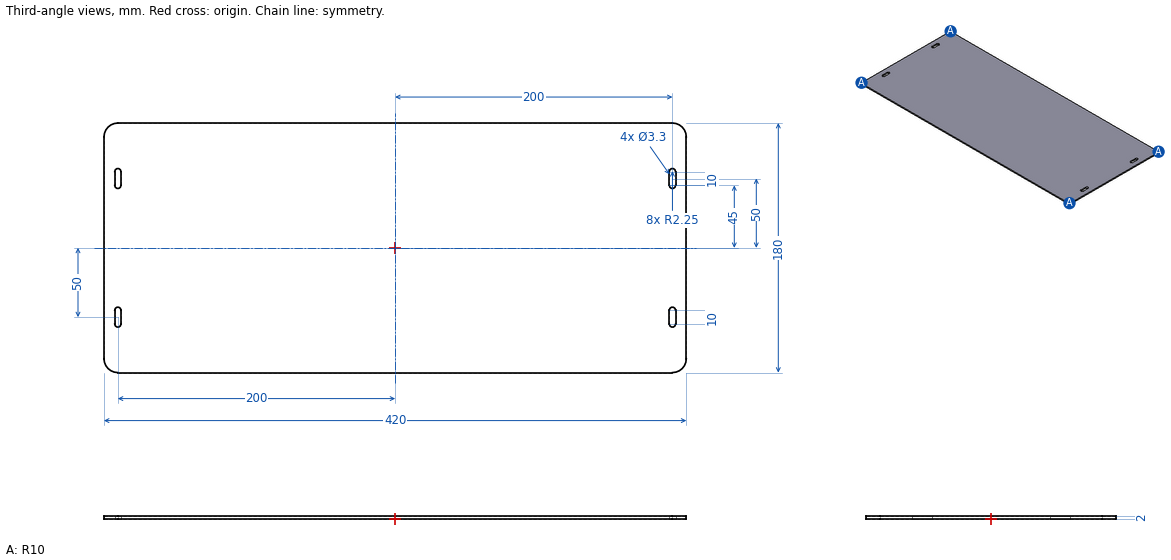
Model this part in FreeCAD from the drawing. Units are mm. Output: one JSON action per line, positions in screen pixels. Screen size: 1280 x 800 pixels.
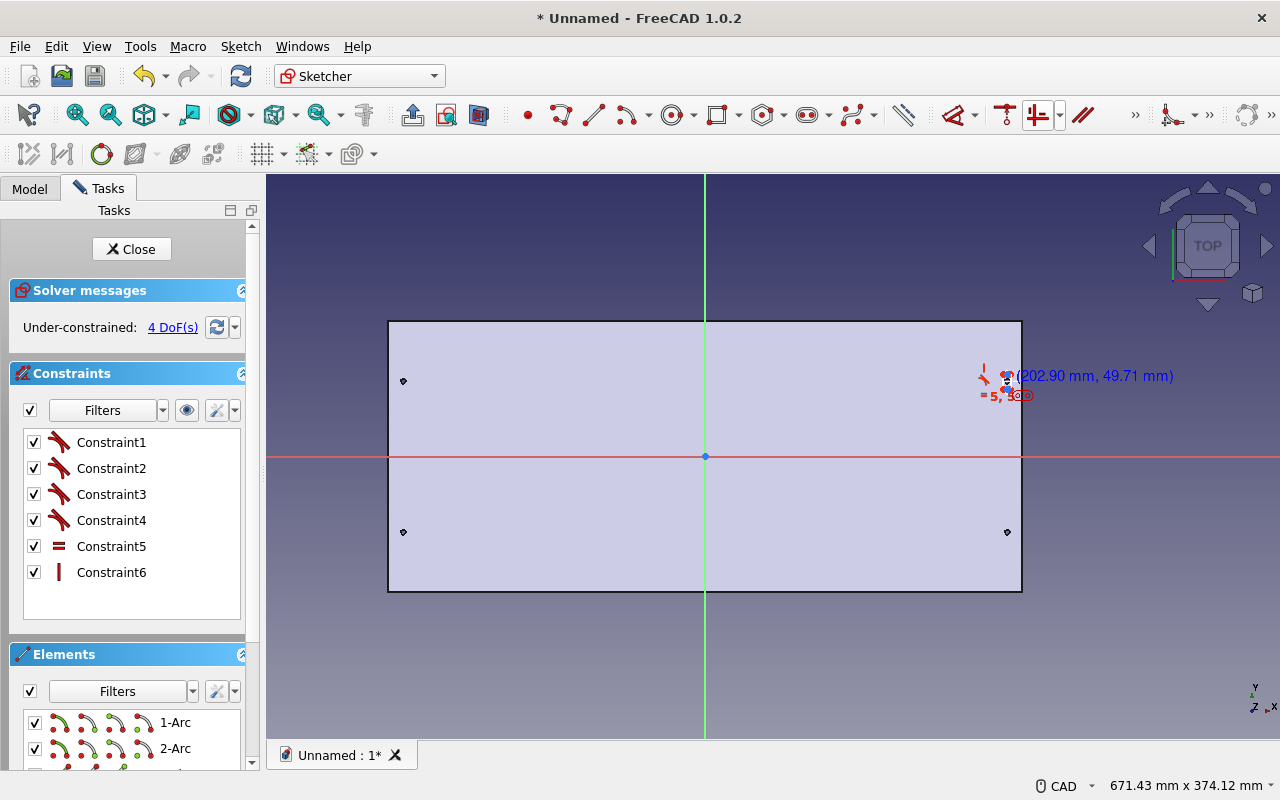
{"action": "scroll", "coordinate": [1007, 540], "scroll_direction": "up", "scroll_amount": 10}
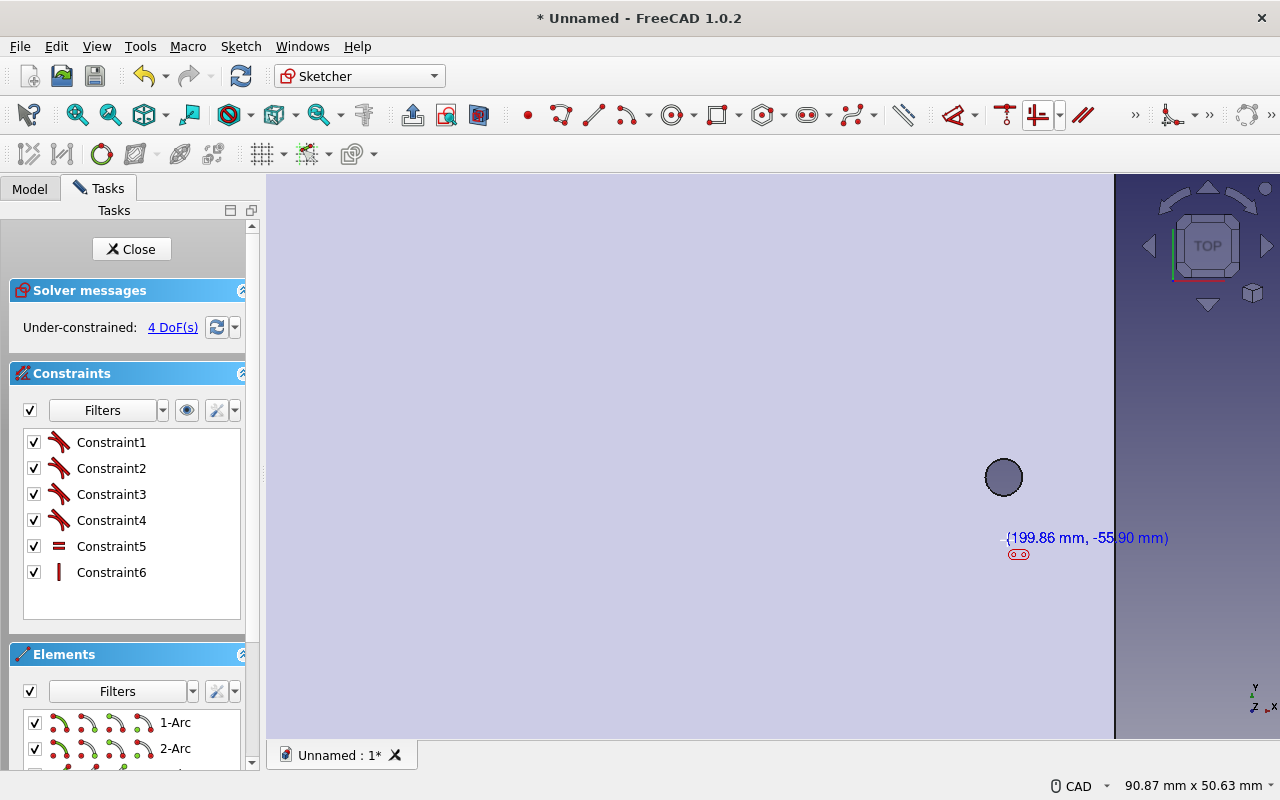
{"action": "scroll", "coordinate": [1007, 541], "scroll_direction": "down", "scroll_amount": 10}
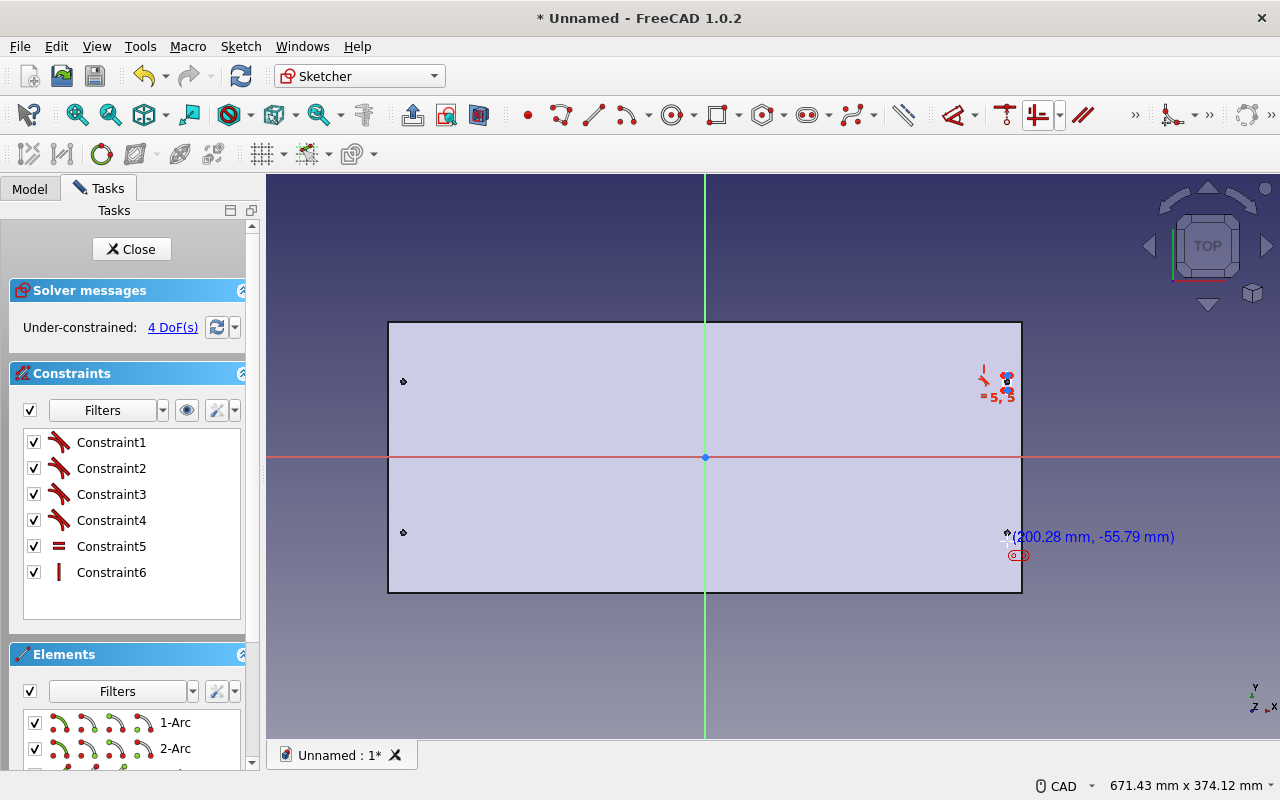
{"action": "left_click", "coordinate": [1007, 540]}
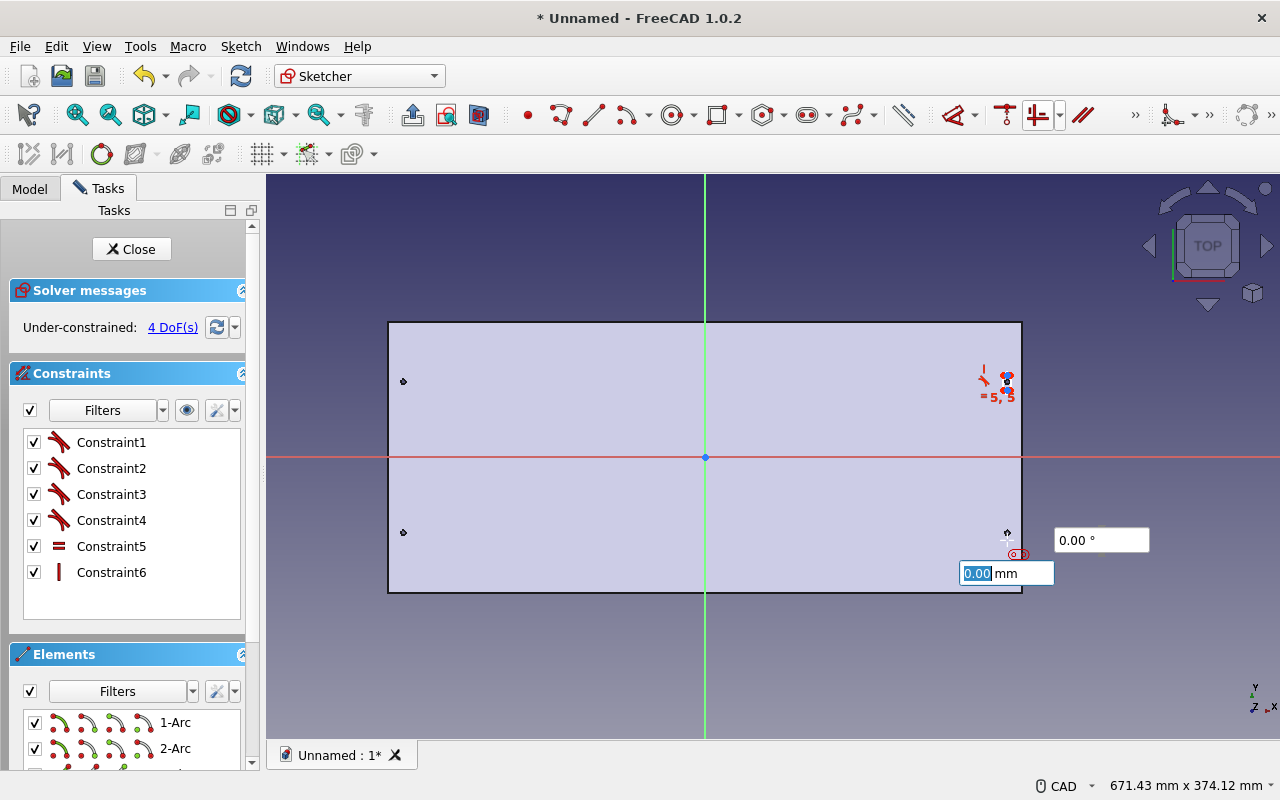
{"action": "left_click", "coordinate": [1007, 525]}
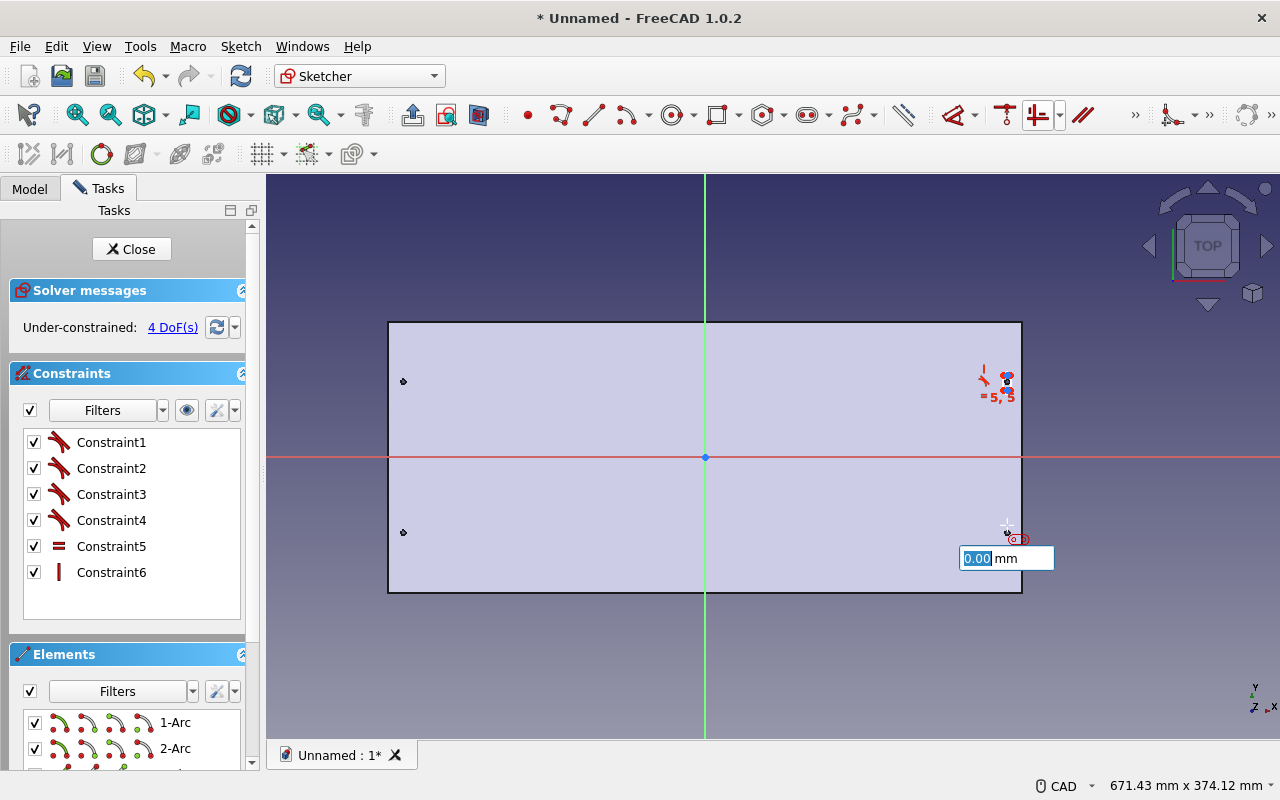
{"action": "scroll", "coordinate": [1004, 533], "scroll_direction": "up", "scroll_amount": 8}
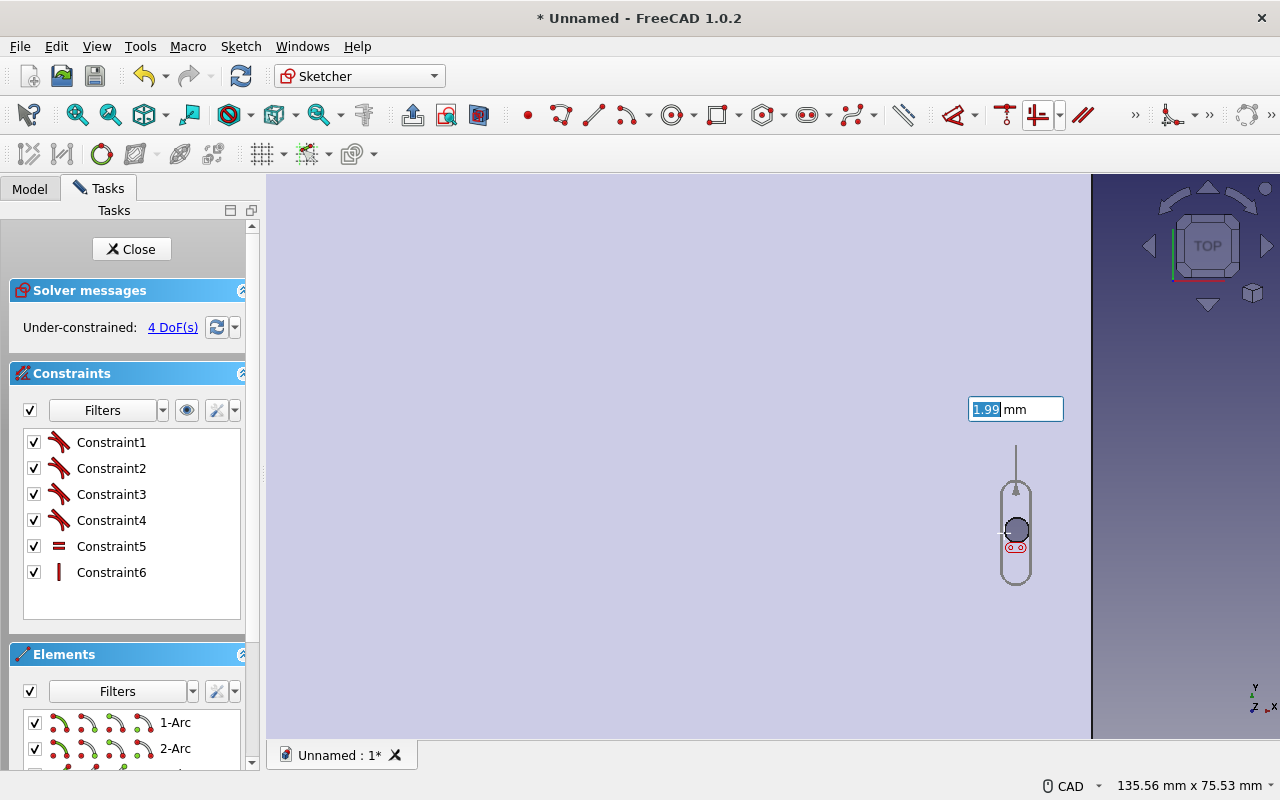
{"action": "left_click", "coordinate": [1000, 530]}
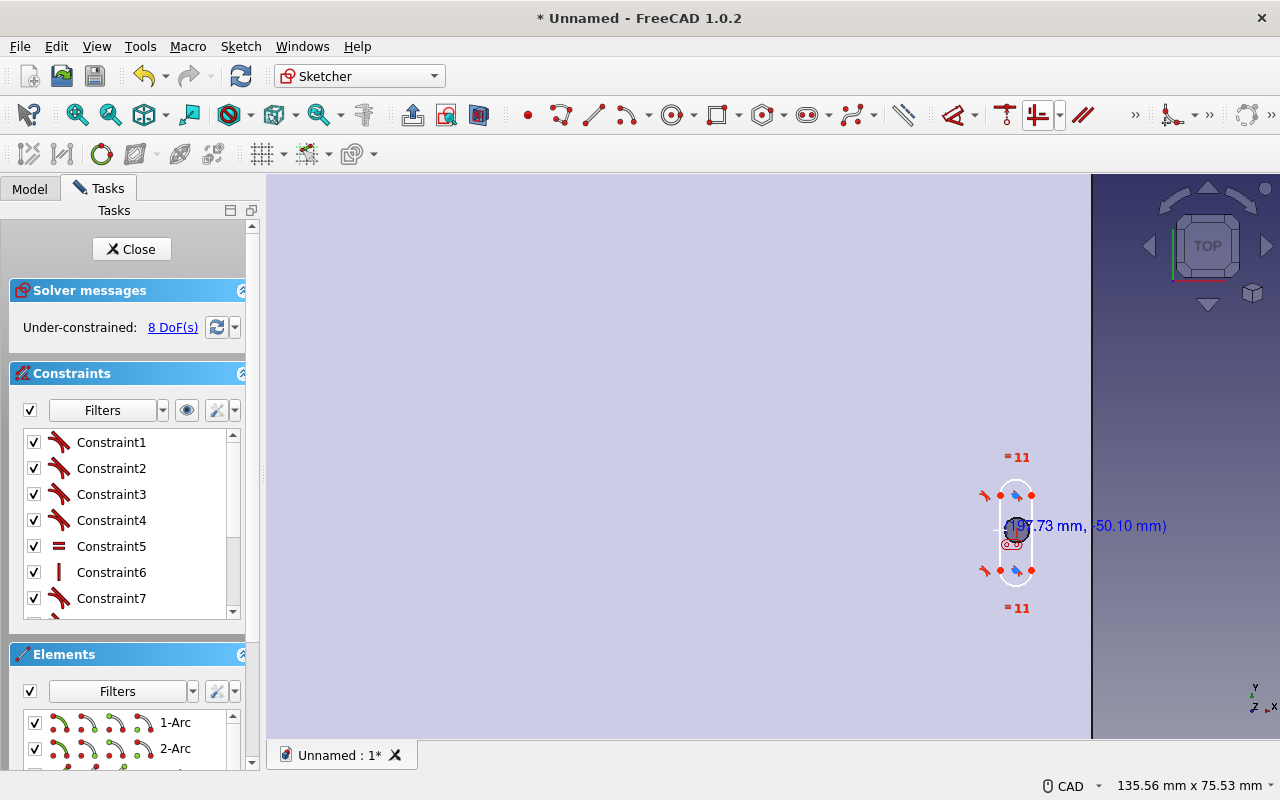
{"action": "scroll", "coordinate": [1004, 532], "scroll_direction": "down", "scroll_amount": 8}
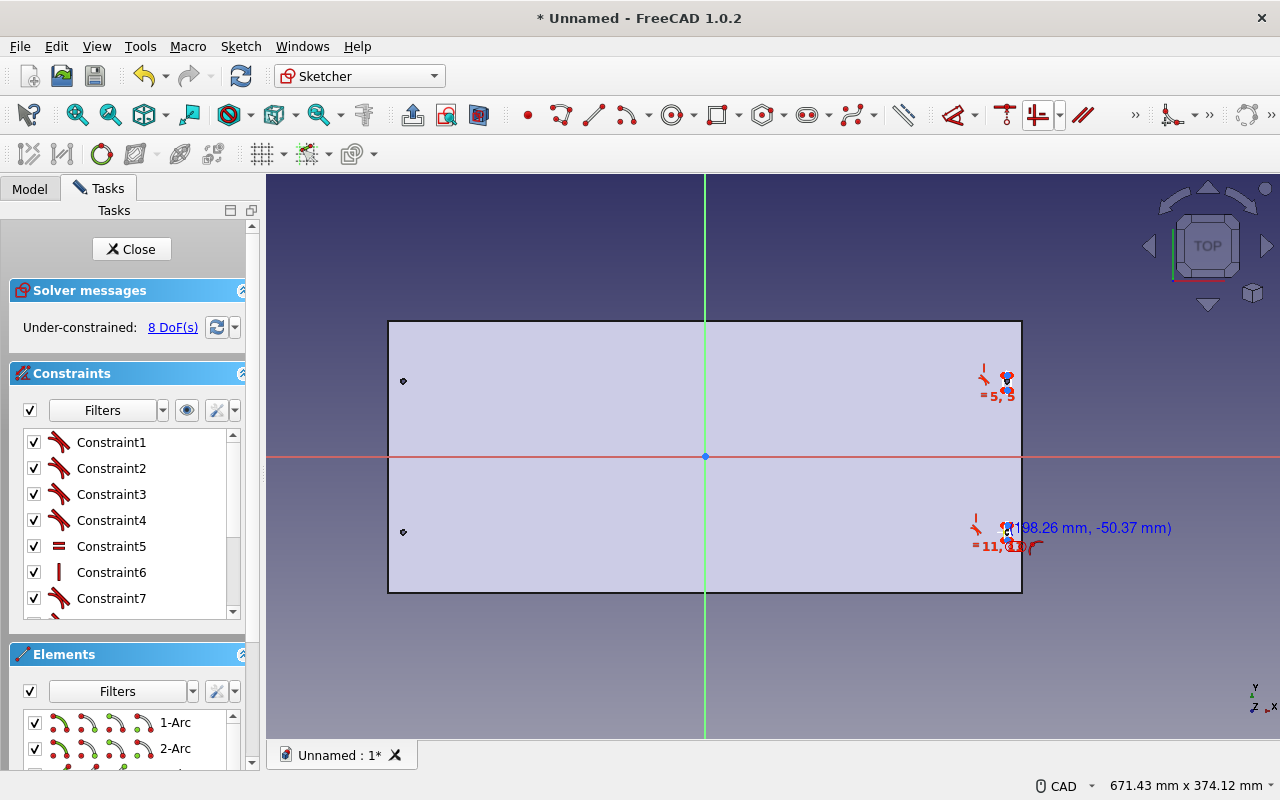
{"action": "scroll", "coordinate": [403, 540], "scroll_direction": "up", "scroll_amount": 10}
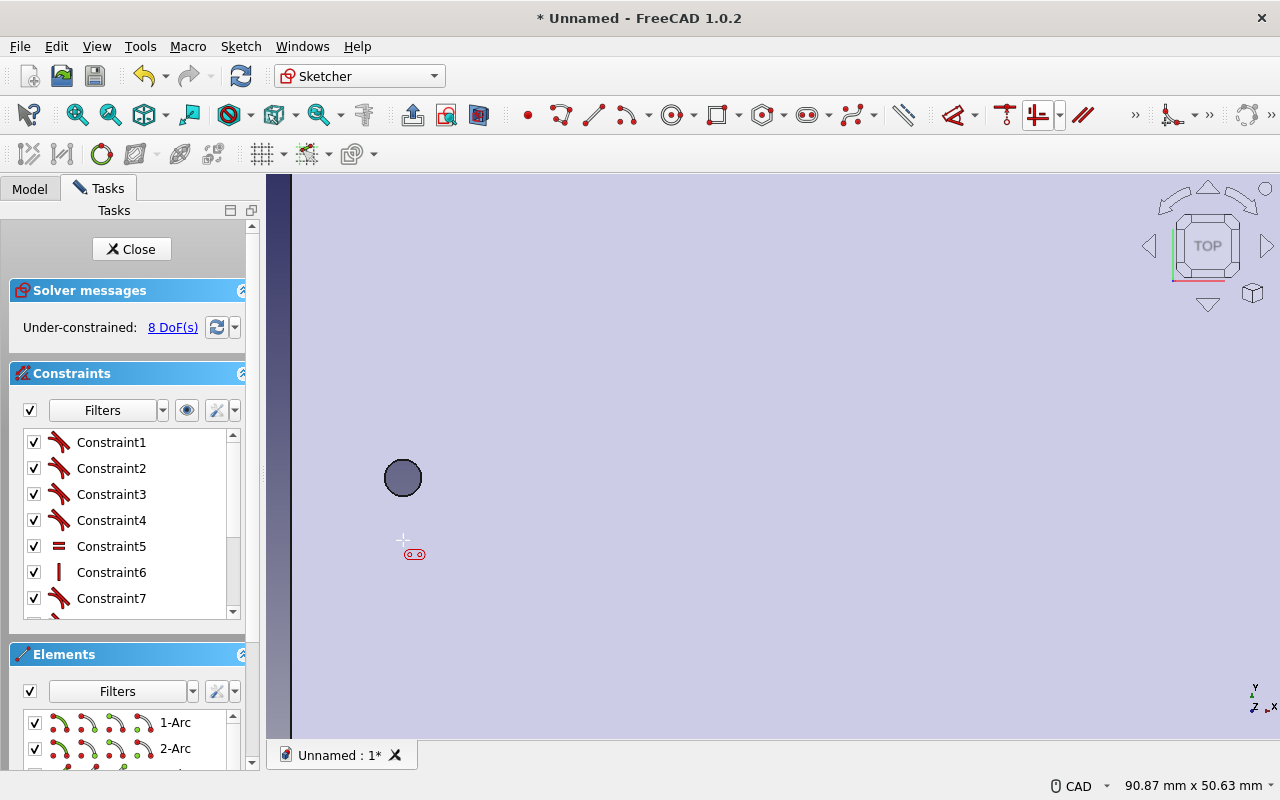
{"action": "scroll", "coordinate": [402, 540], "scroll_direction": "down", "scroll_amount": 10}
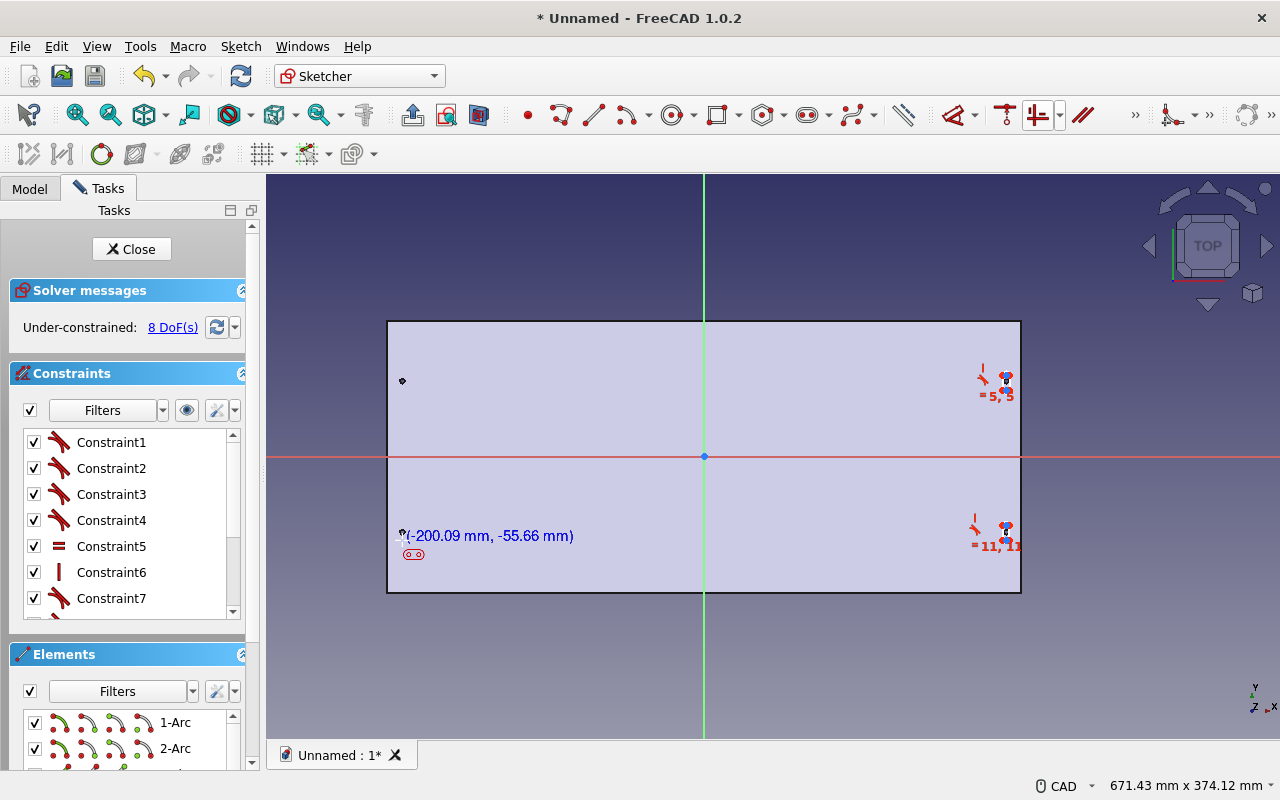
{"action": "left_click", "coordinate": [402, 540]}